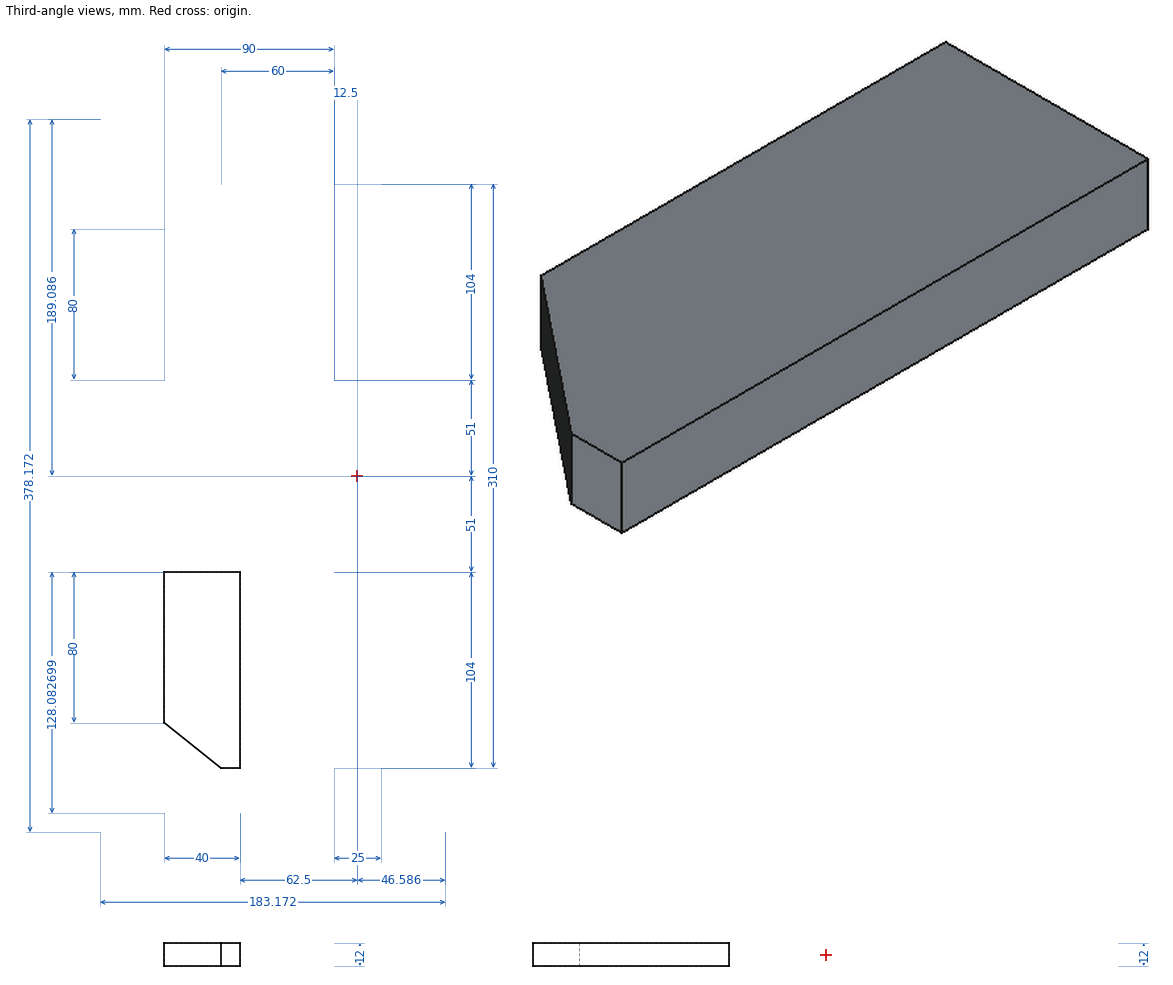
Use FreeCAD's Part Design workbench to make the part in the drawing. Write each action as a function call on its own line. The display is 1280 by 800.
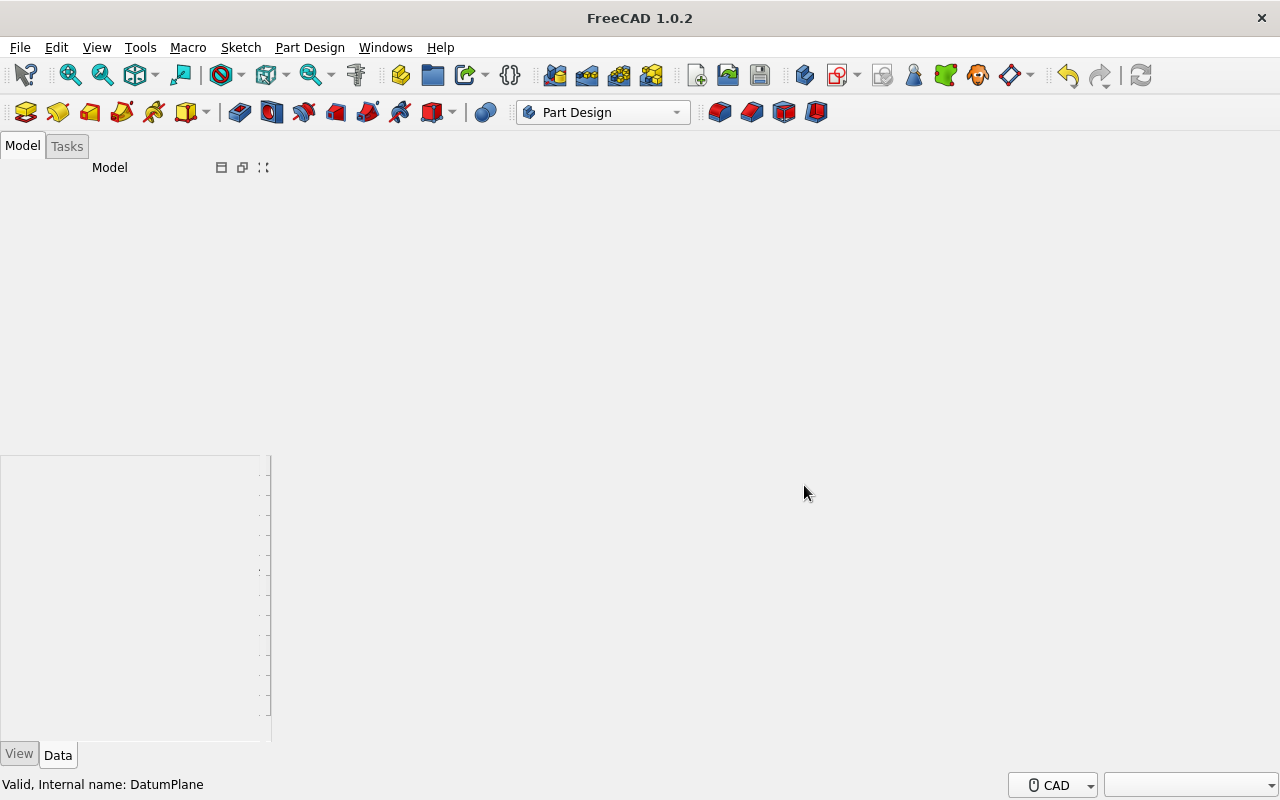
click(696, 76)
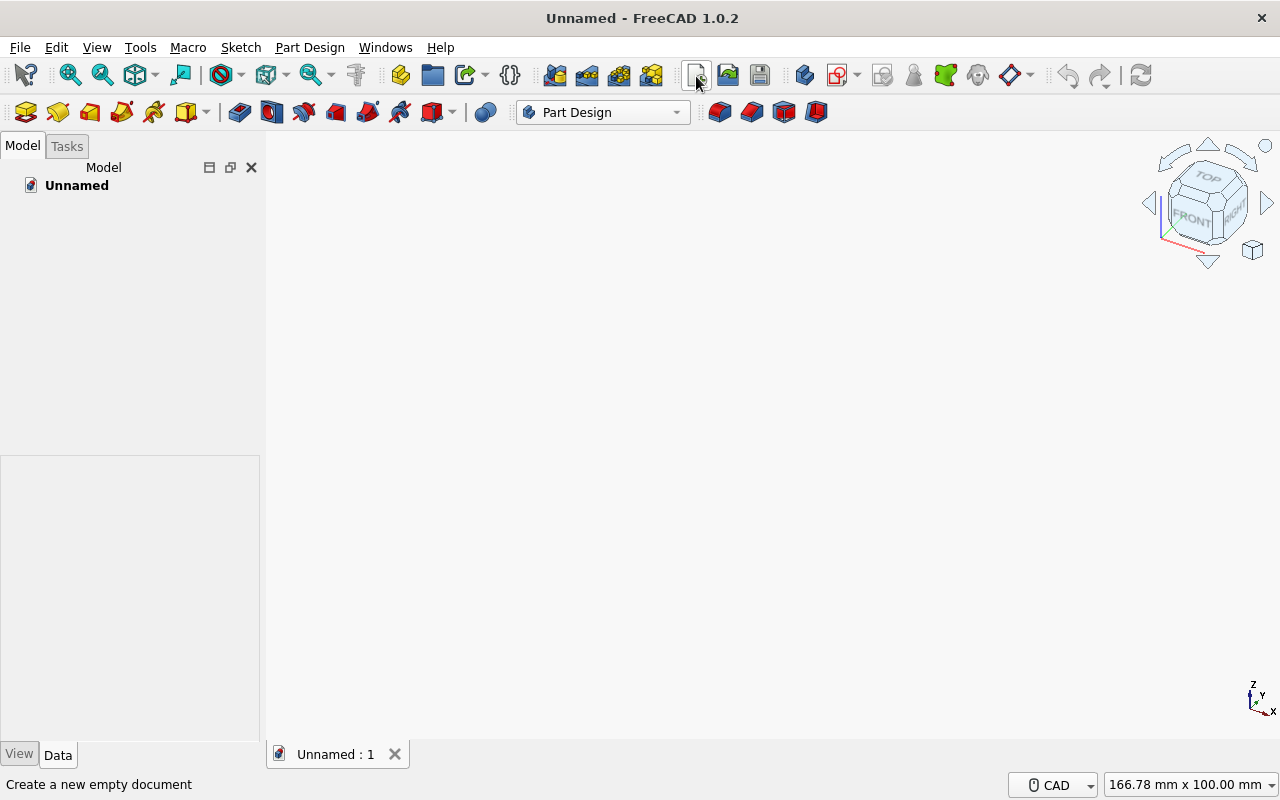
click(838, 76)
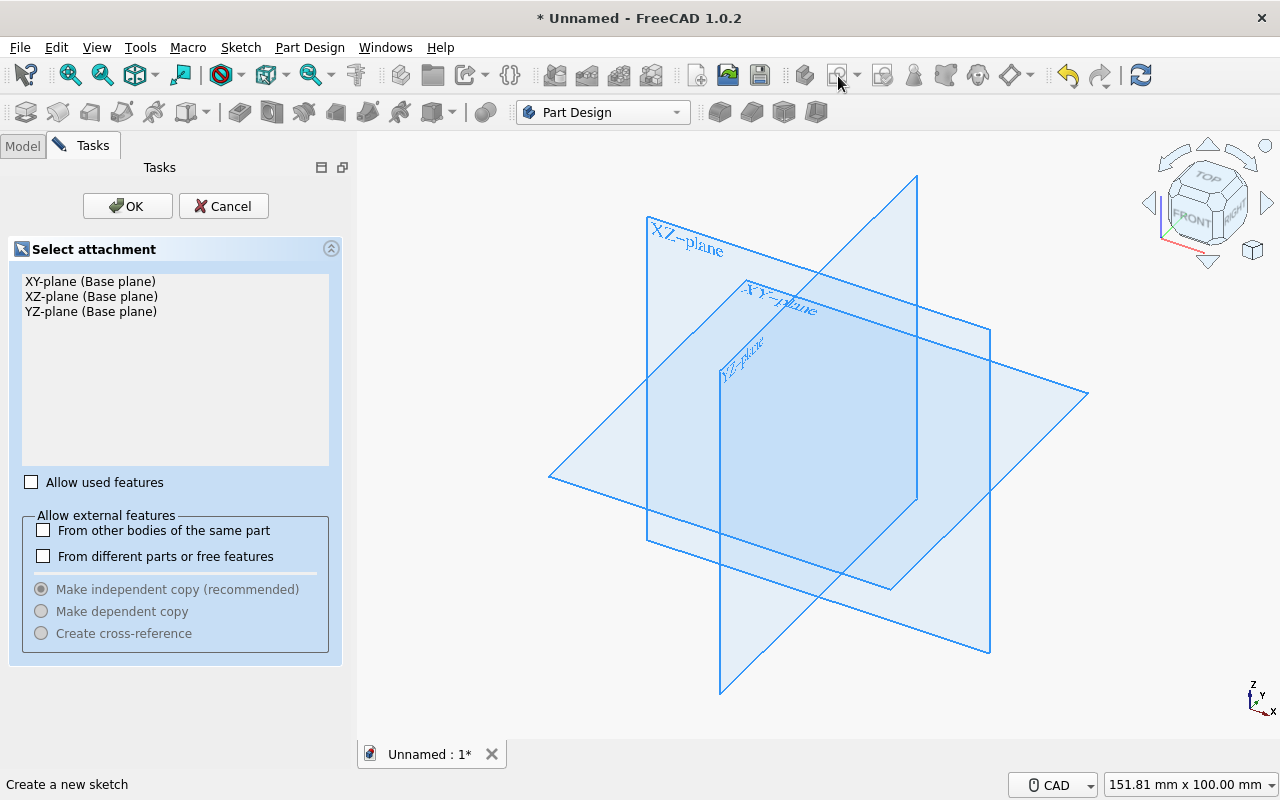
click(82, 282)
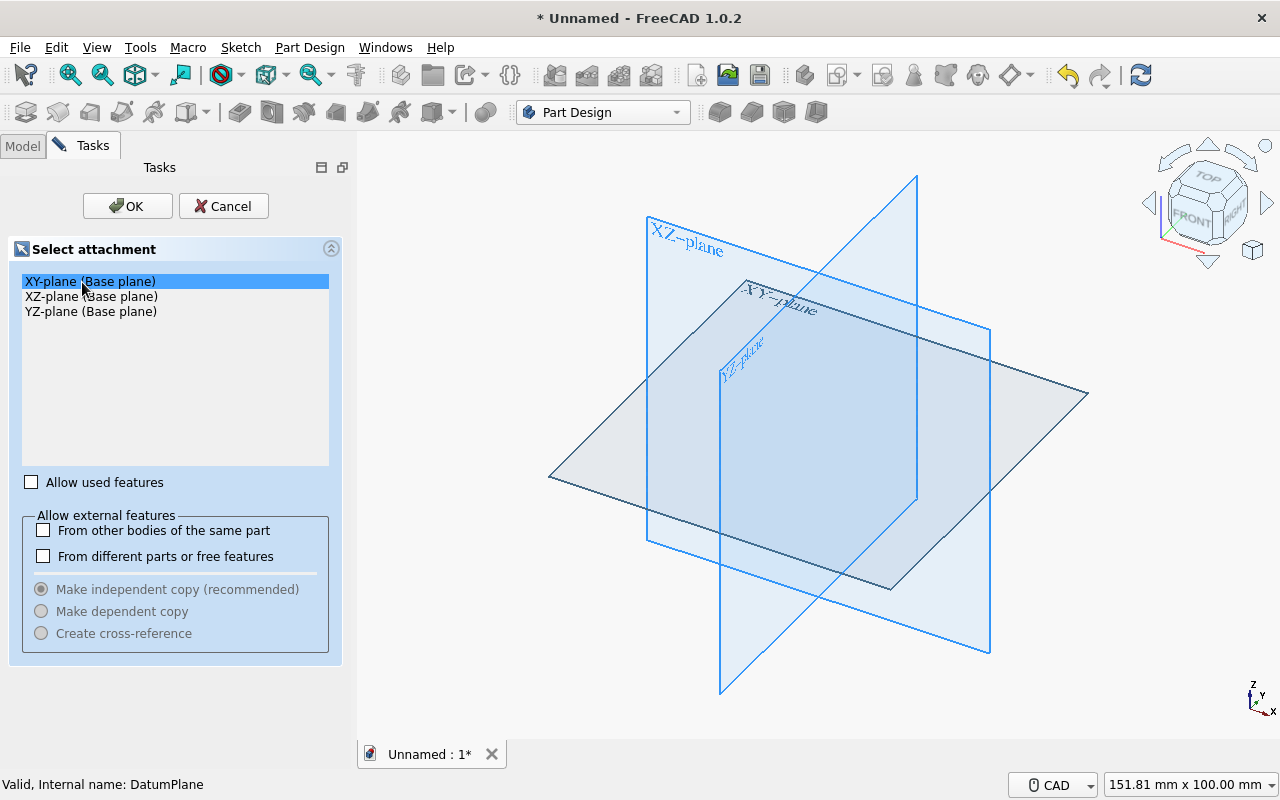
click(128, 206)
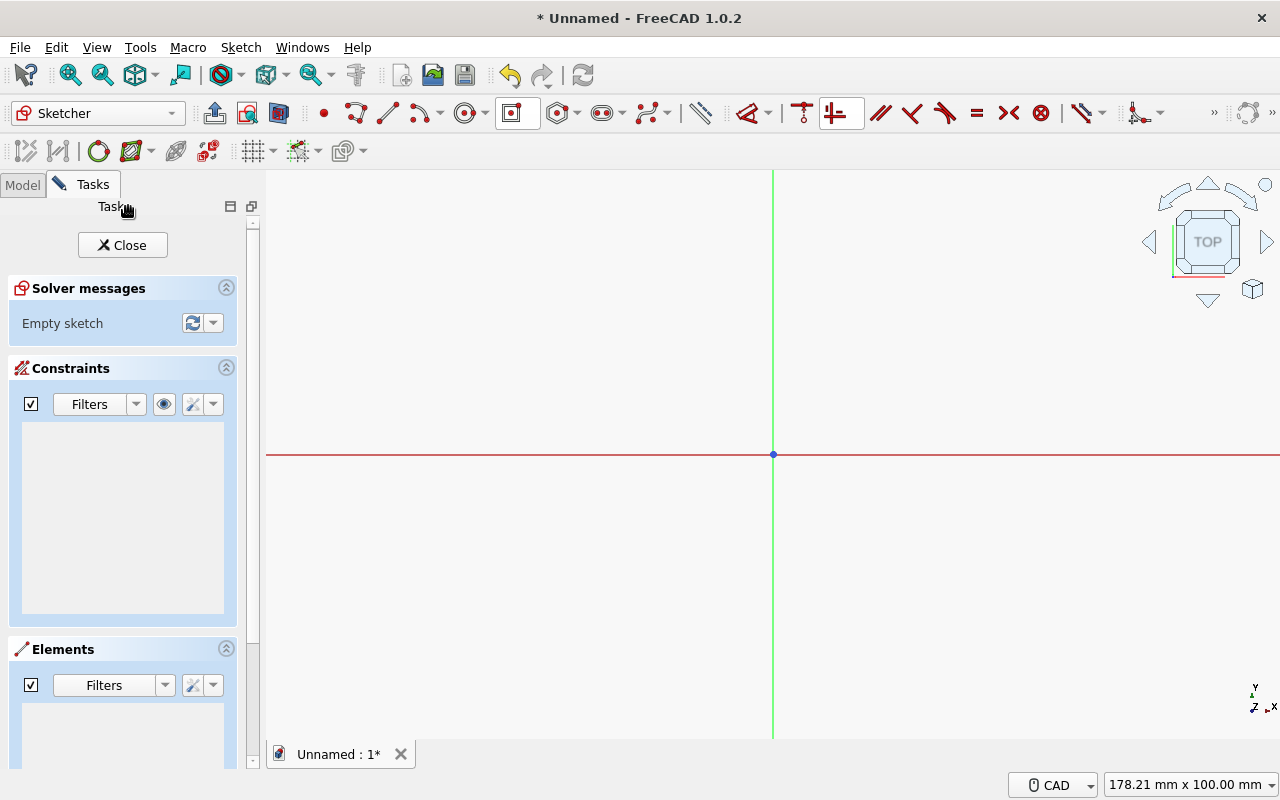
scroll(687, 454, down, 8)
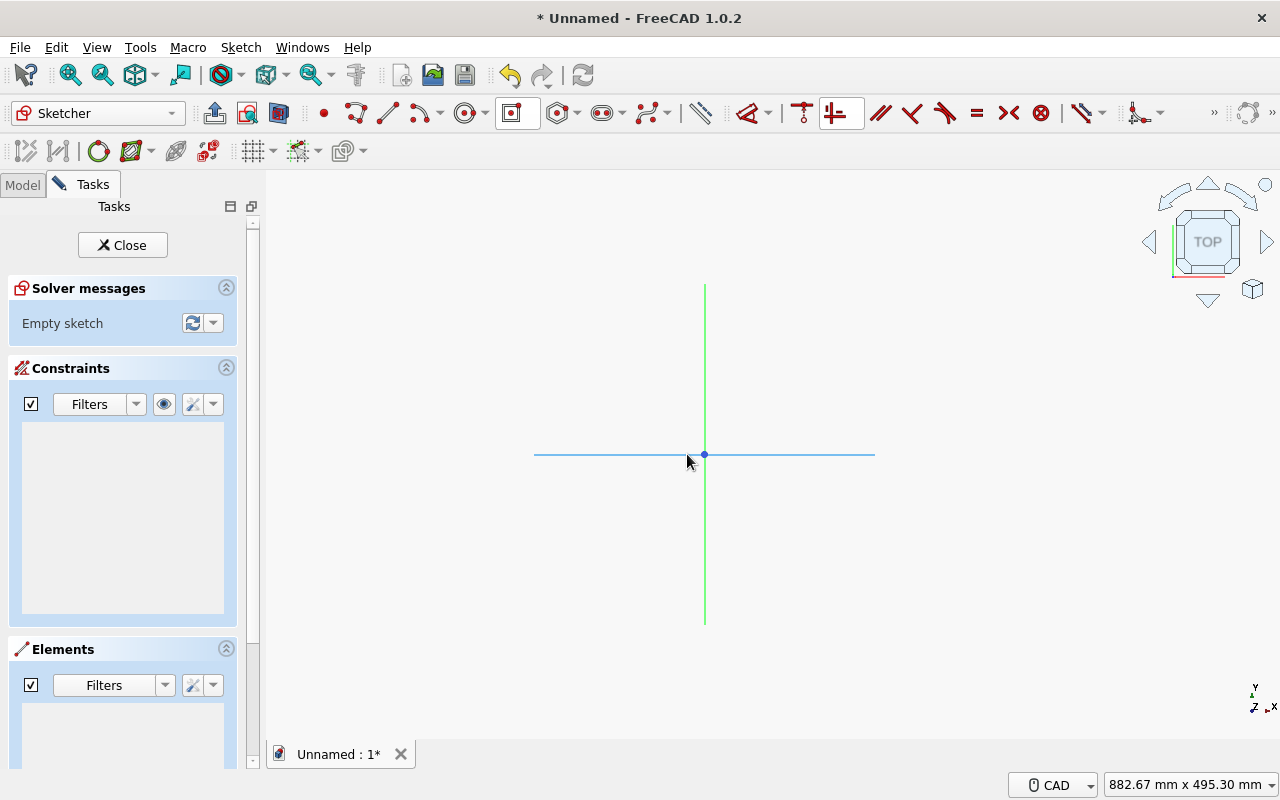
click(512, 114)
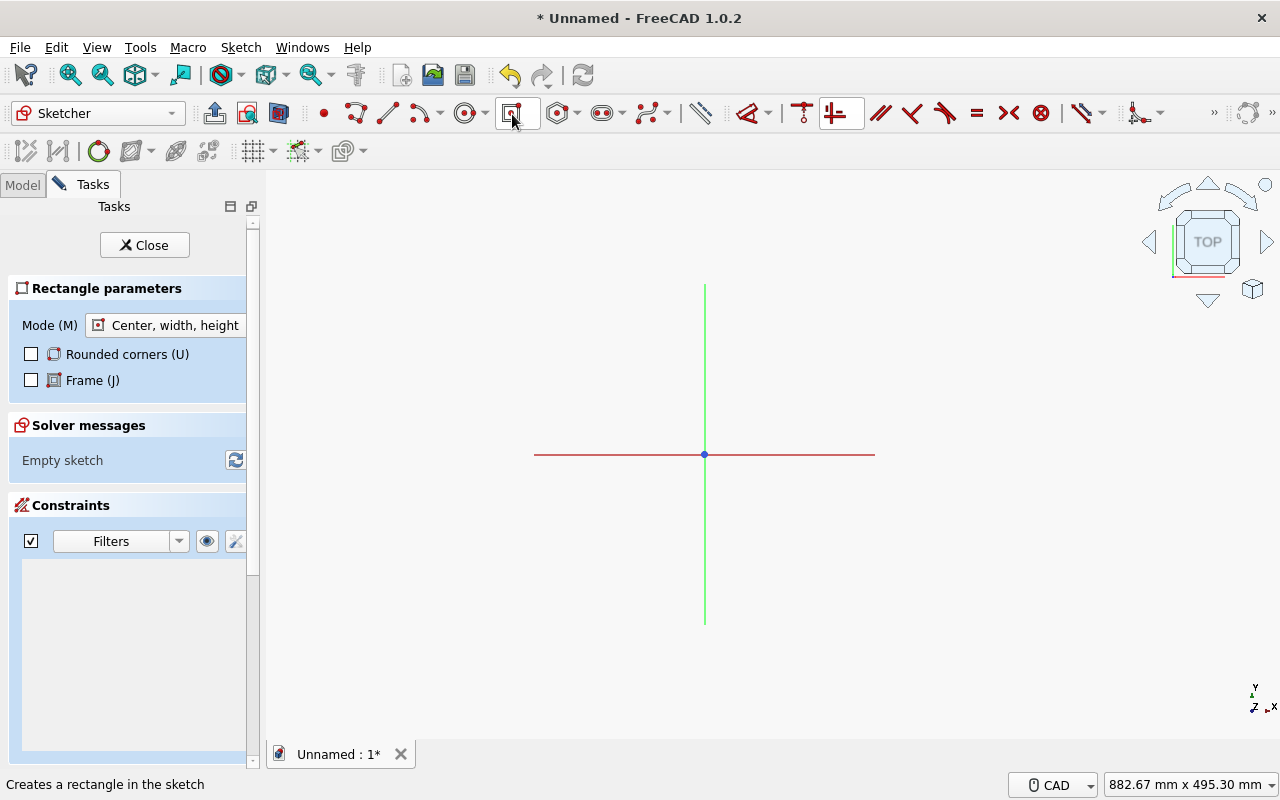
click(705, 454)
click(719, 276)
key(Escape)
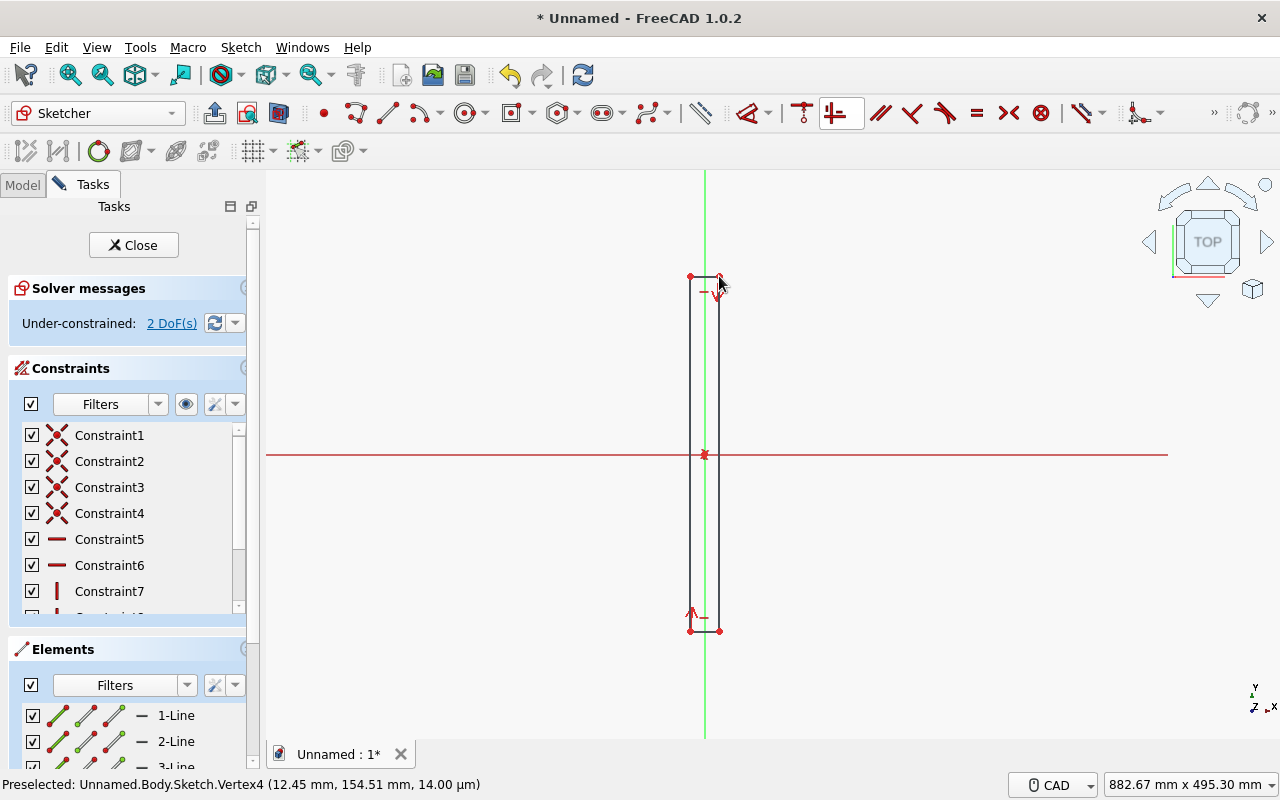
scroll(702, 632, up, 2)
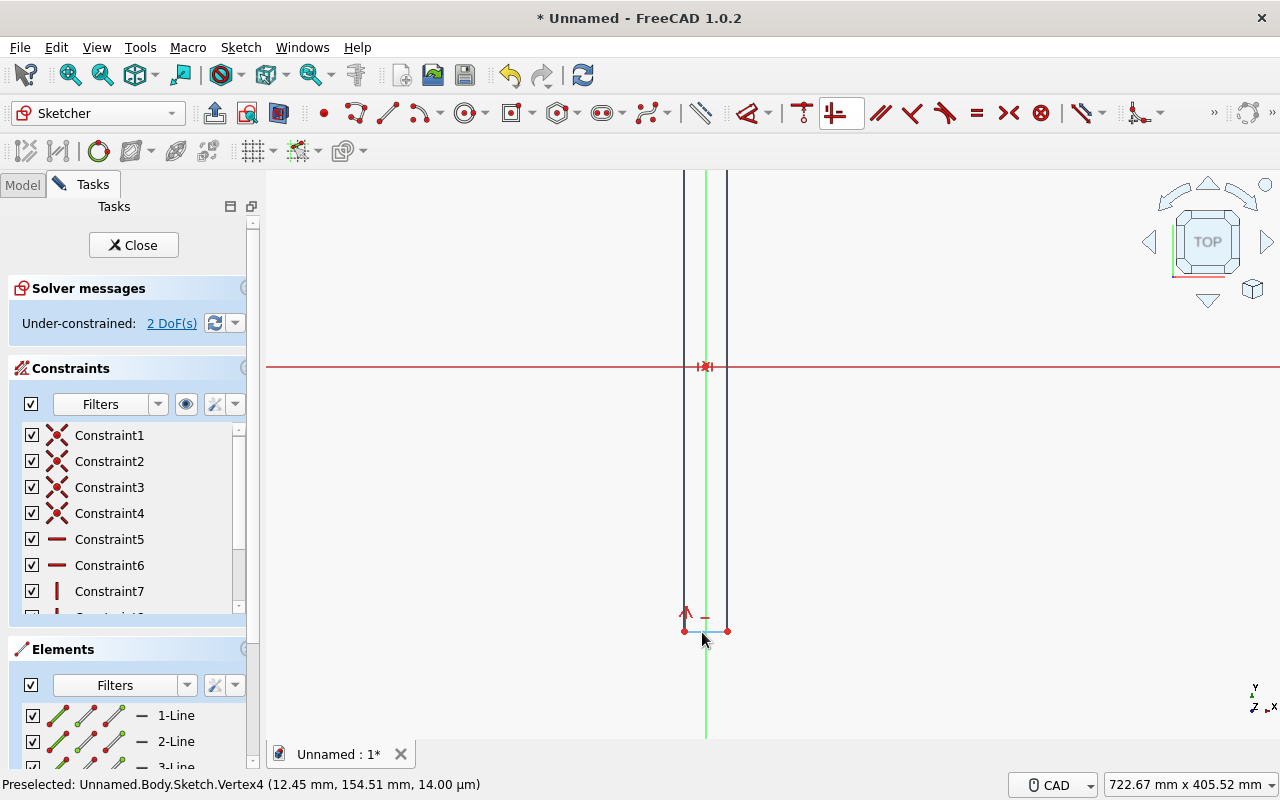
click(702, 632)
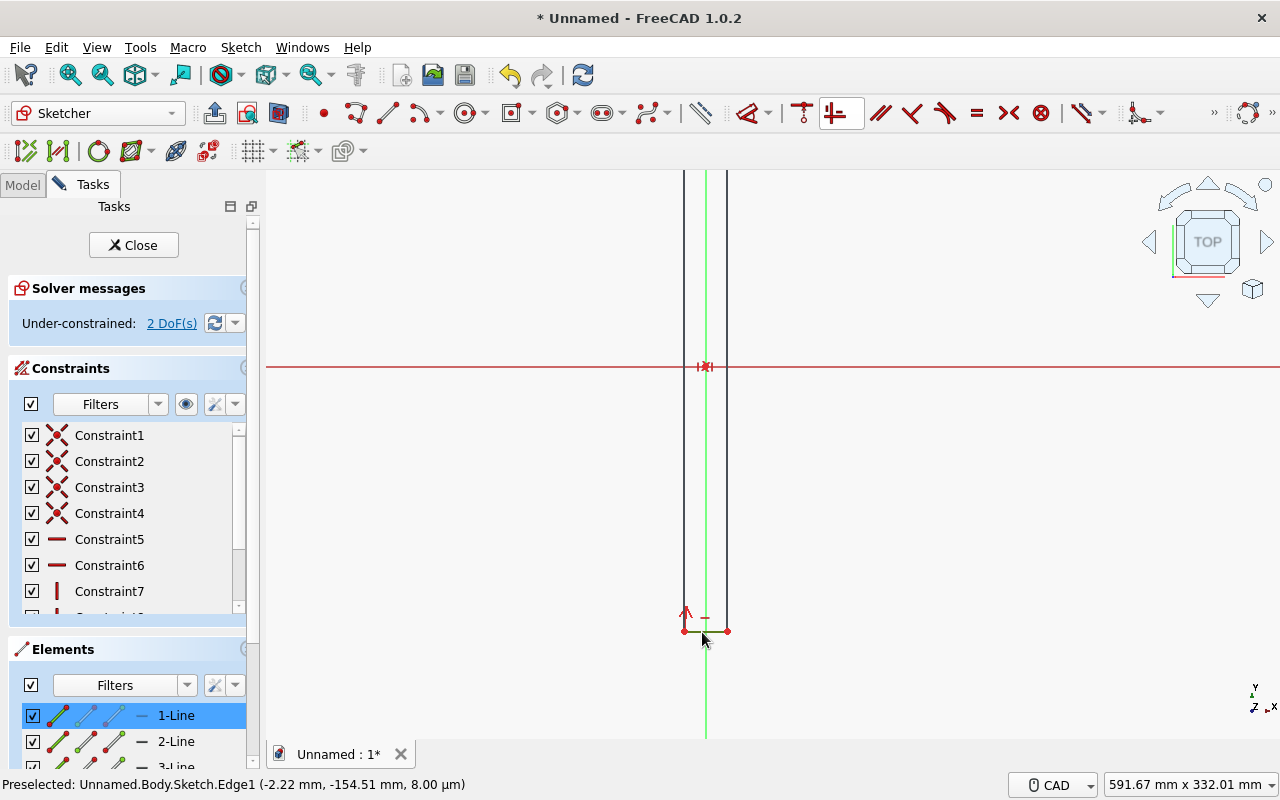
click(770, 114)